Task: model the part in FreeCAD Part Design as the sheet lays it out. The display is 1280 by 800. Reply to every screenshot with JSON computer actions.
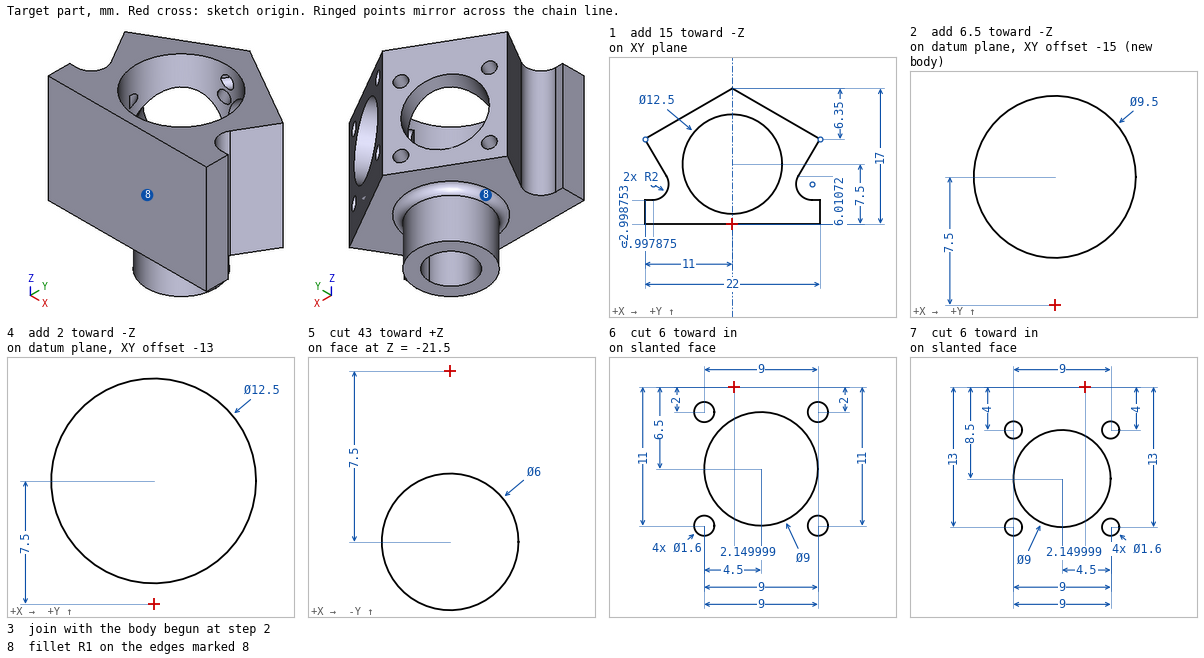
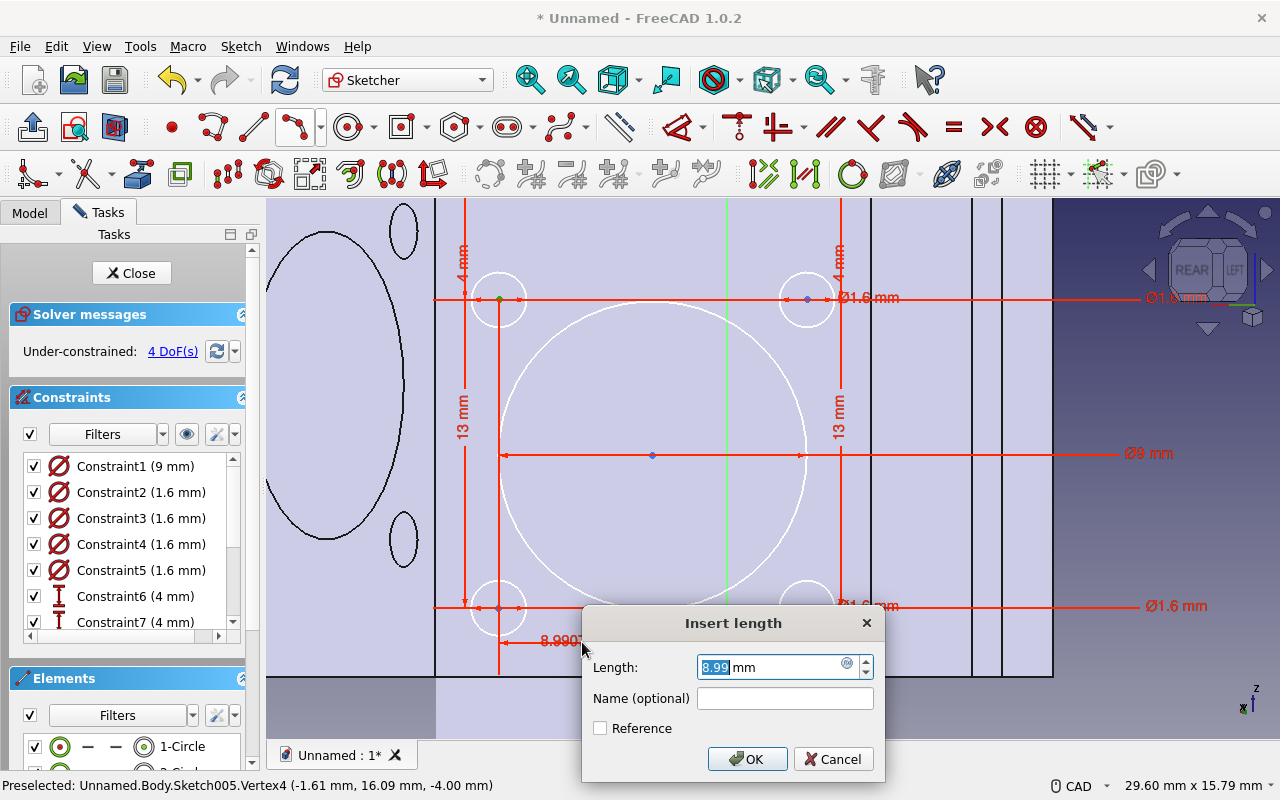
{"action": "type", "text": "9"}
{"action": "key", "text": "Return"}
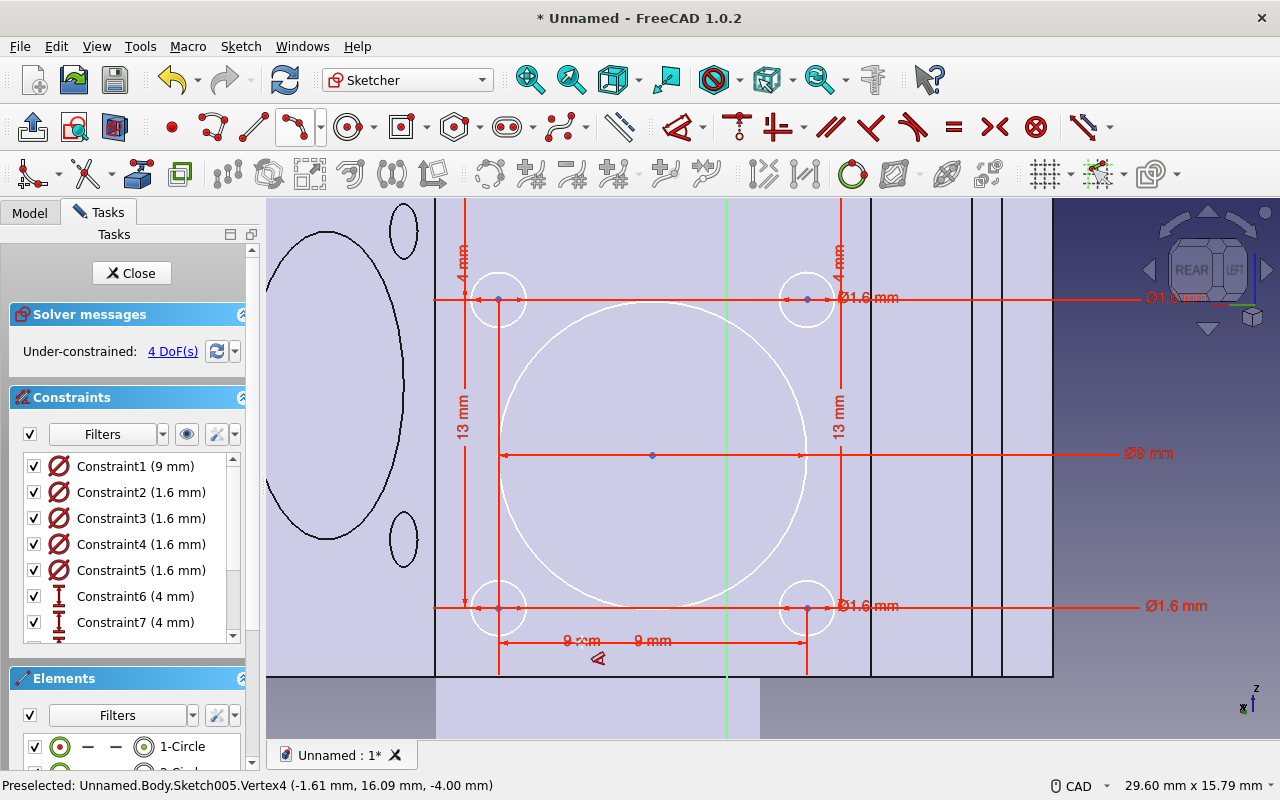
{"action": "left_click", "coordinate": [499, 300]}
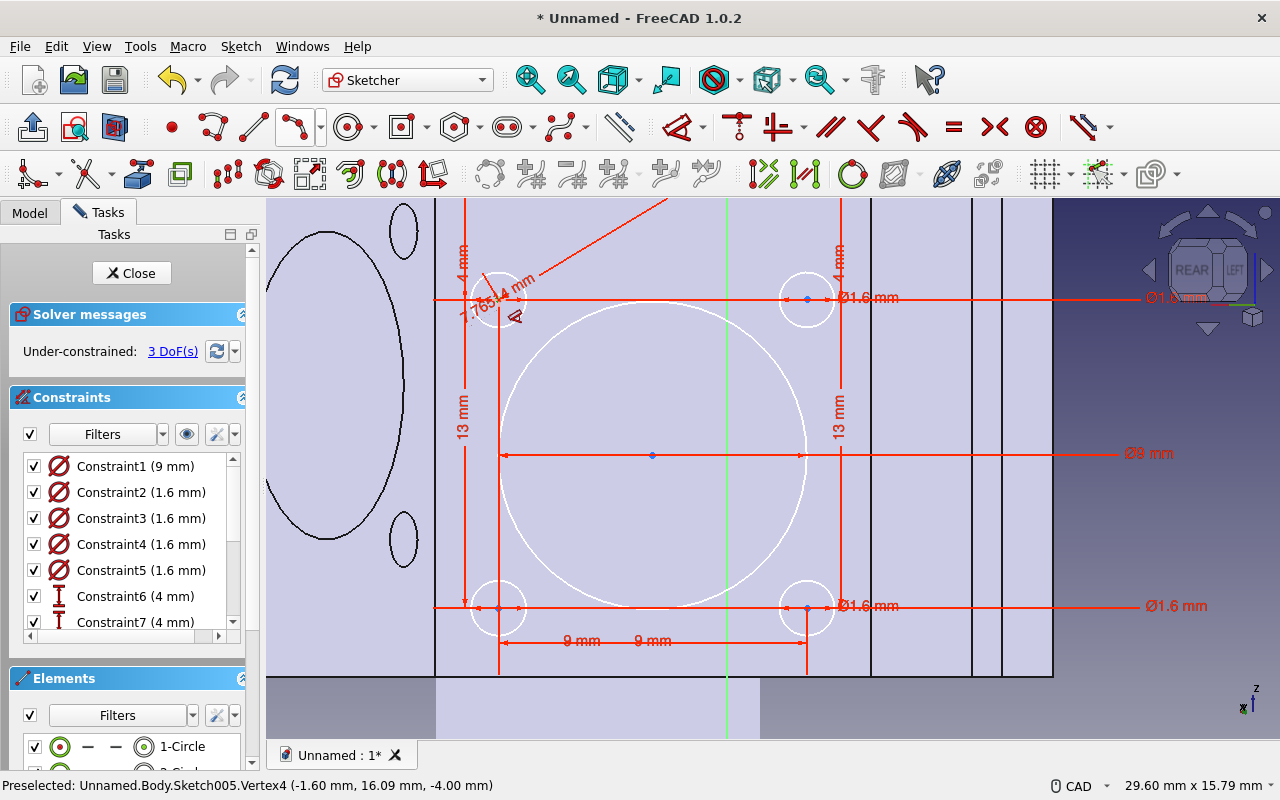
{"action": "left_click", "coordinate": [807, 300]}
{"action": "left_click", "coordinate": [653, 266]}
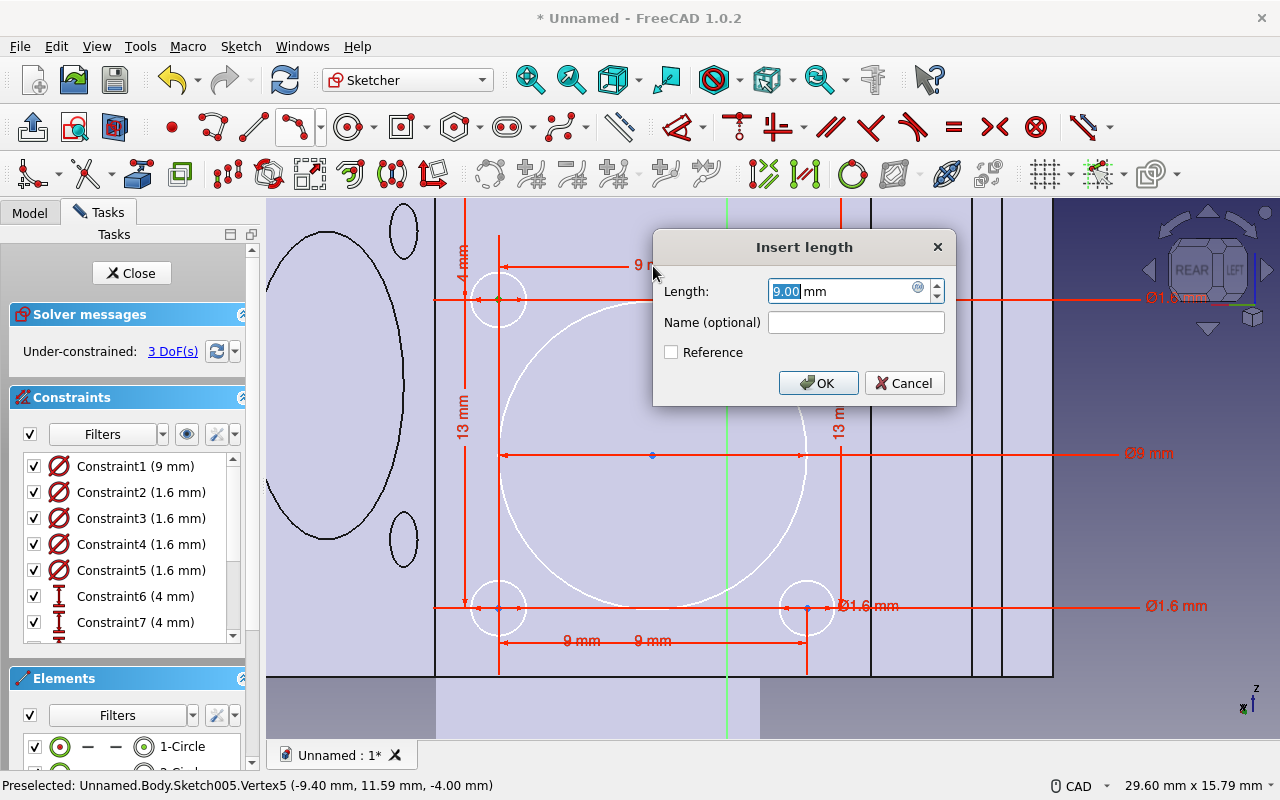
{"action": "type", "text": "9"}
{"action": "key", "text": "Return"}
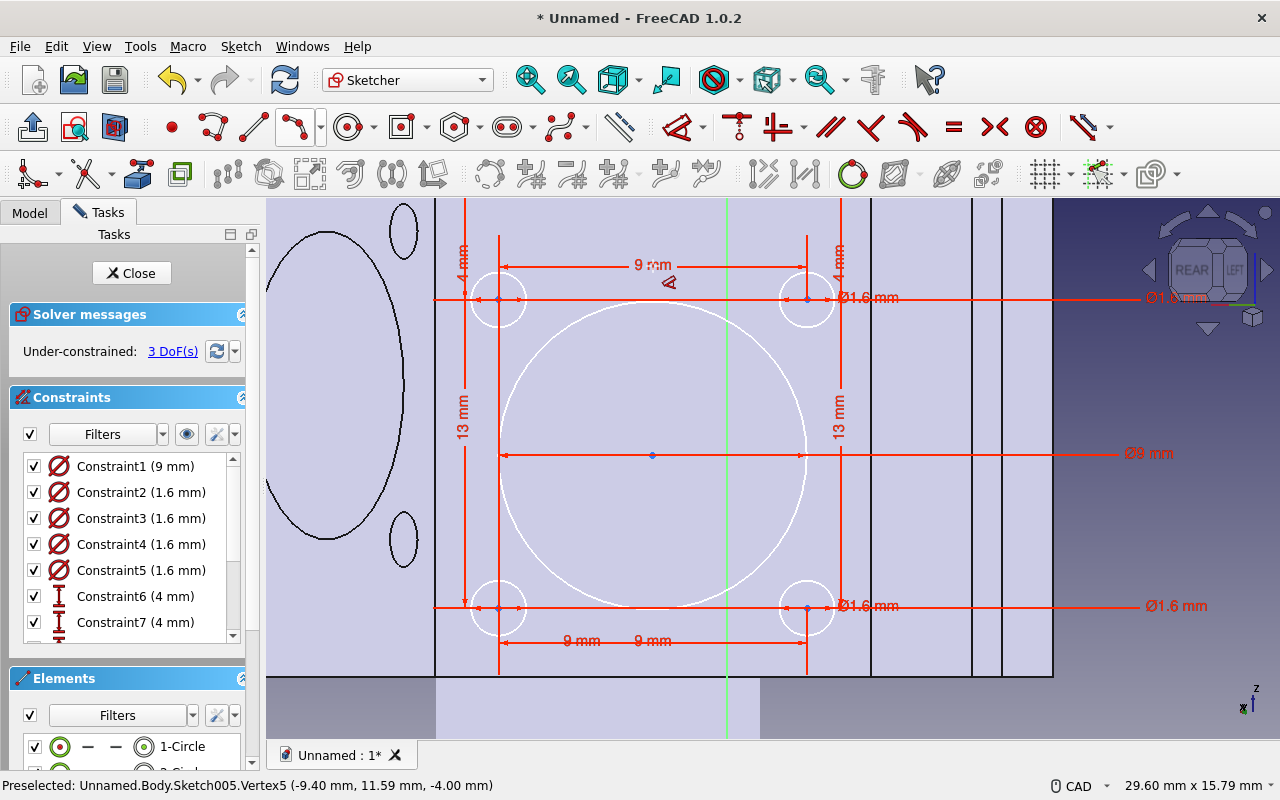
{"action": "left_click", "coordinate": [653, 455]}
{"action": "left_click", "coordinate": [761, 288]}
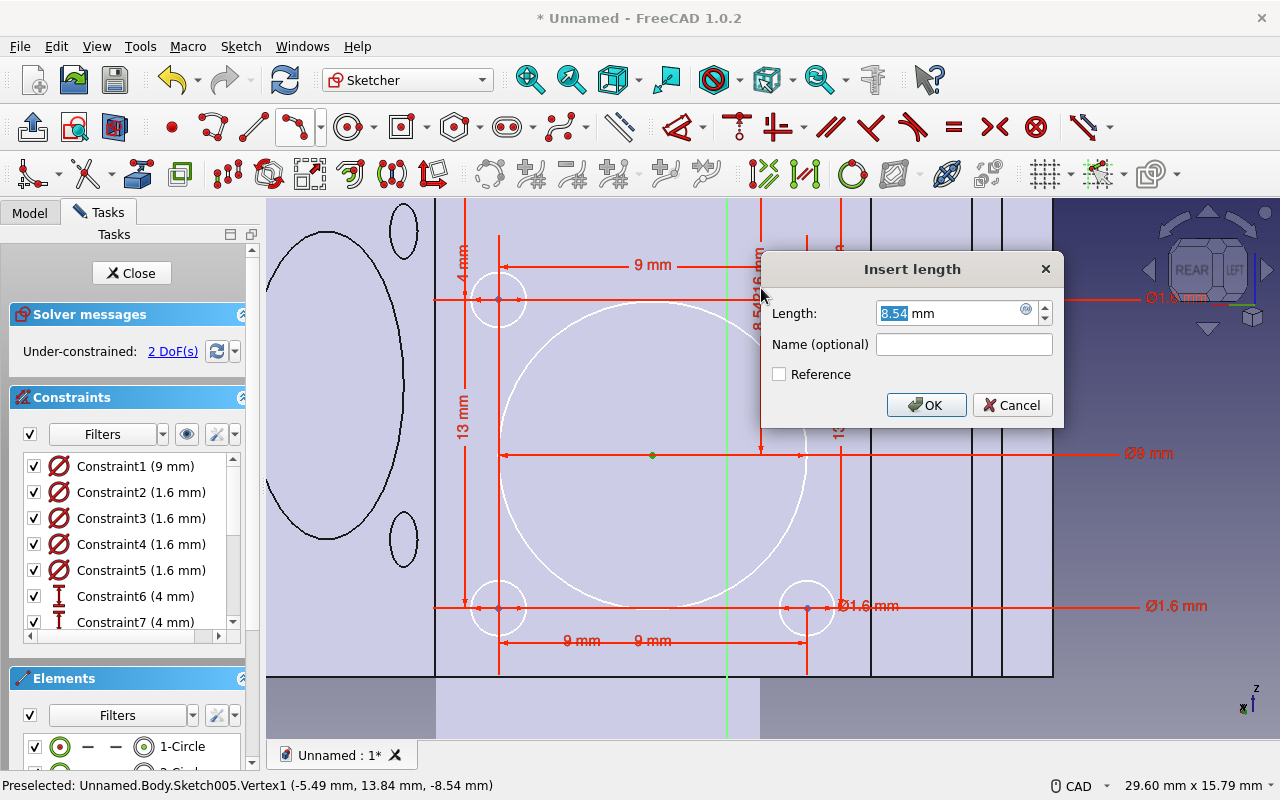
{"action": "type", "text": "8.5"}
{"action": "key", "text": "Return"}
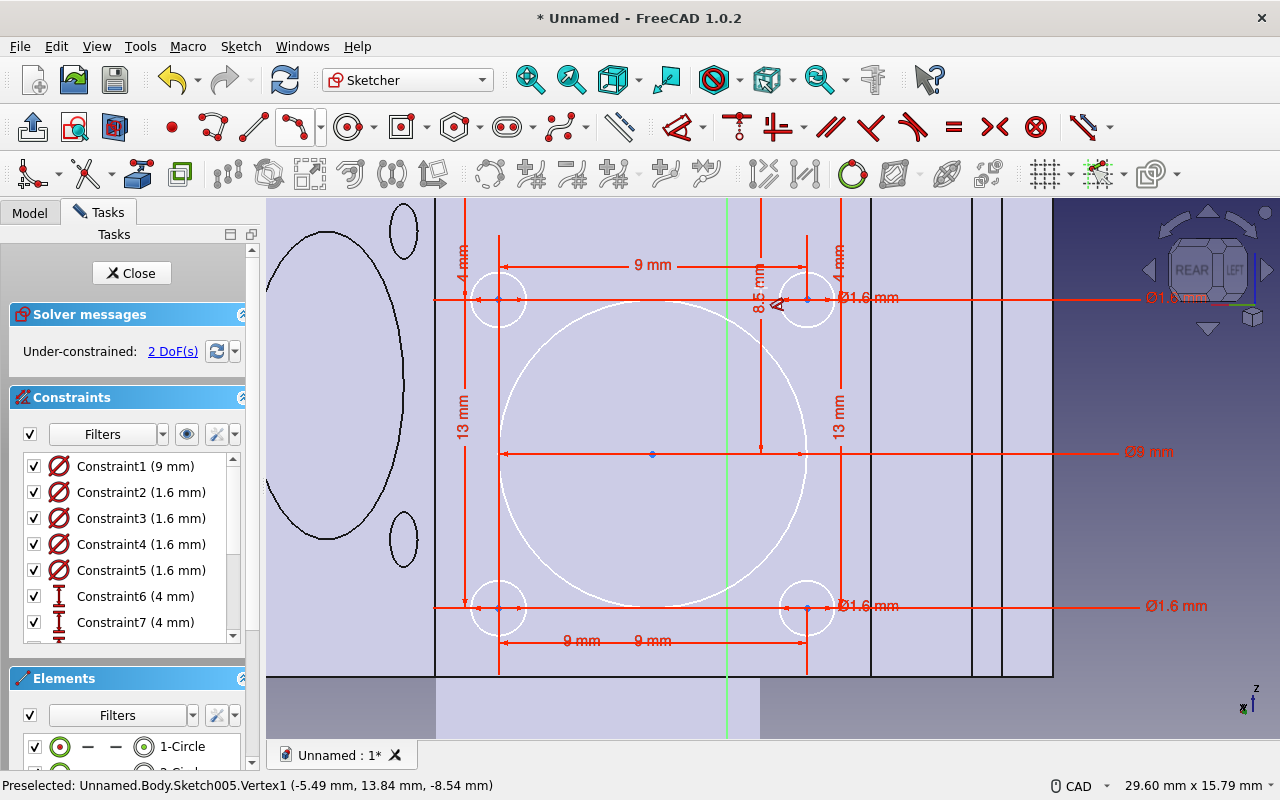
{"action": "left_click", "coordinate": [653, 454]}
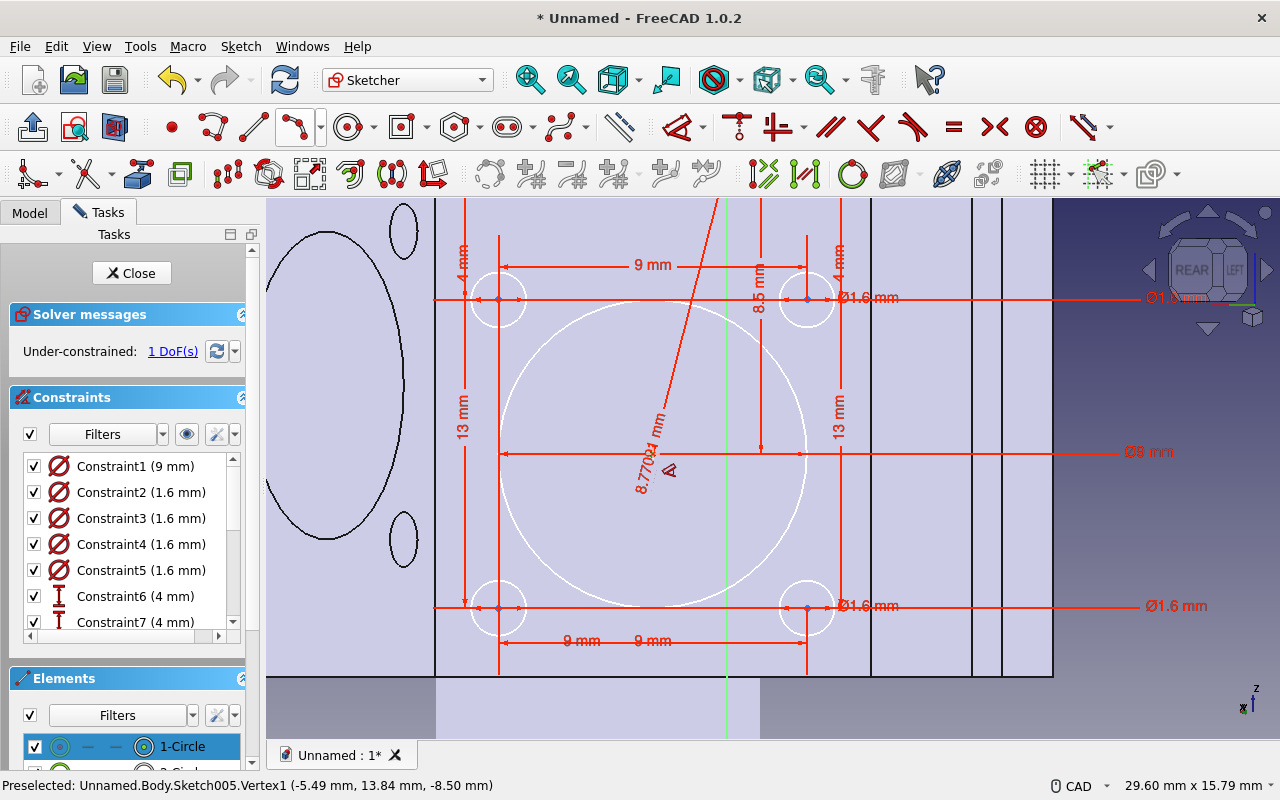
{"action": "left_click", "coordinate": [807, 608]}
{"action": "left_click", "coordinate": [765, 642]}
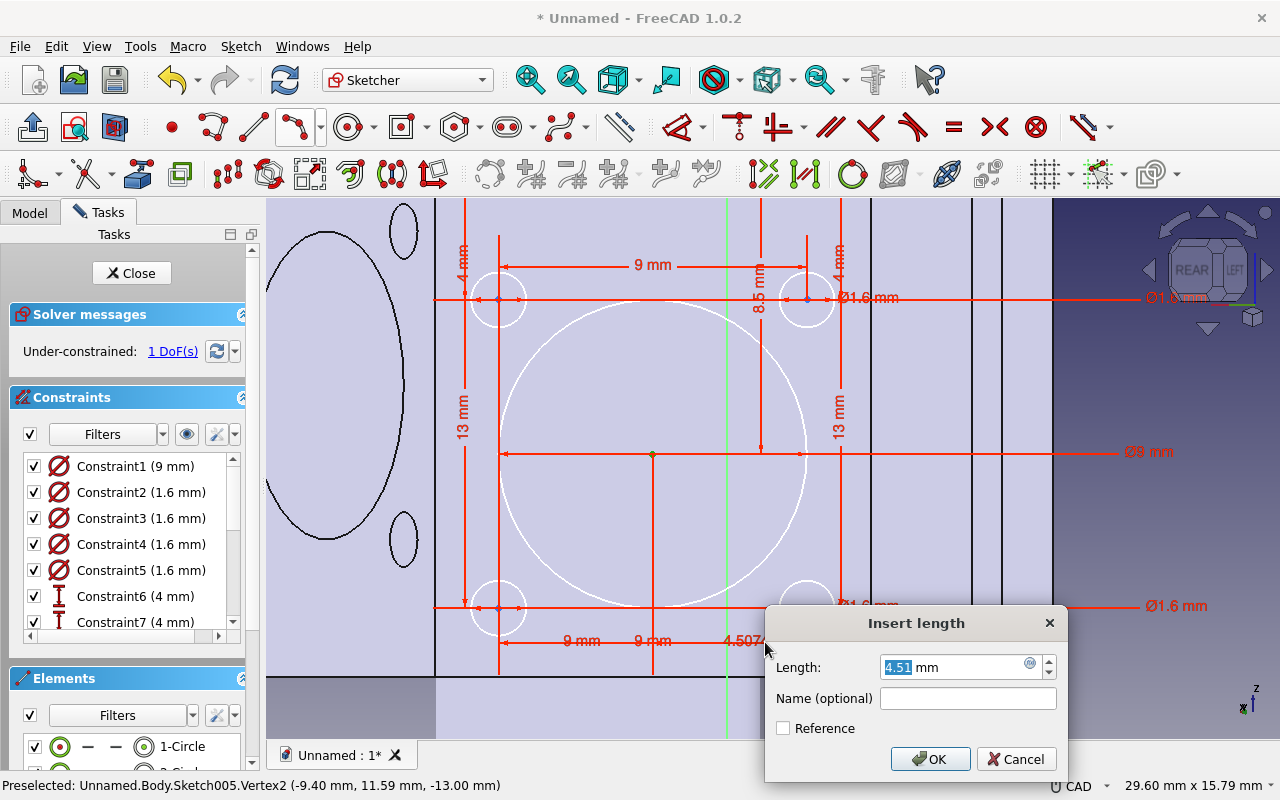
{"action": "type", "text": "4.5"}
{"action": "key", "text": "Return"}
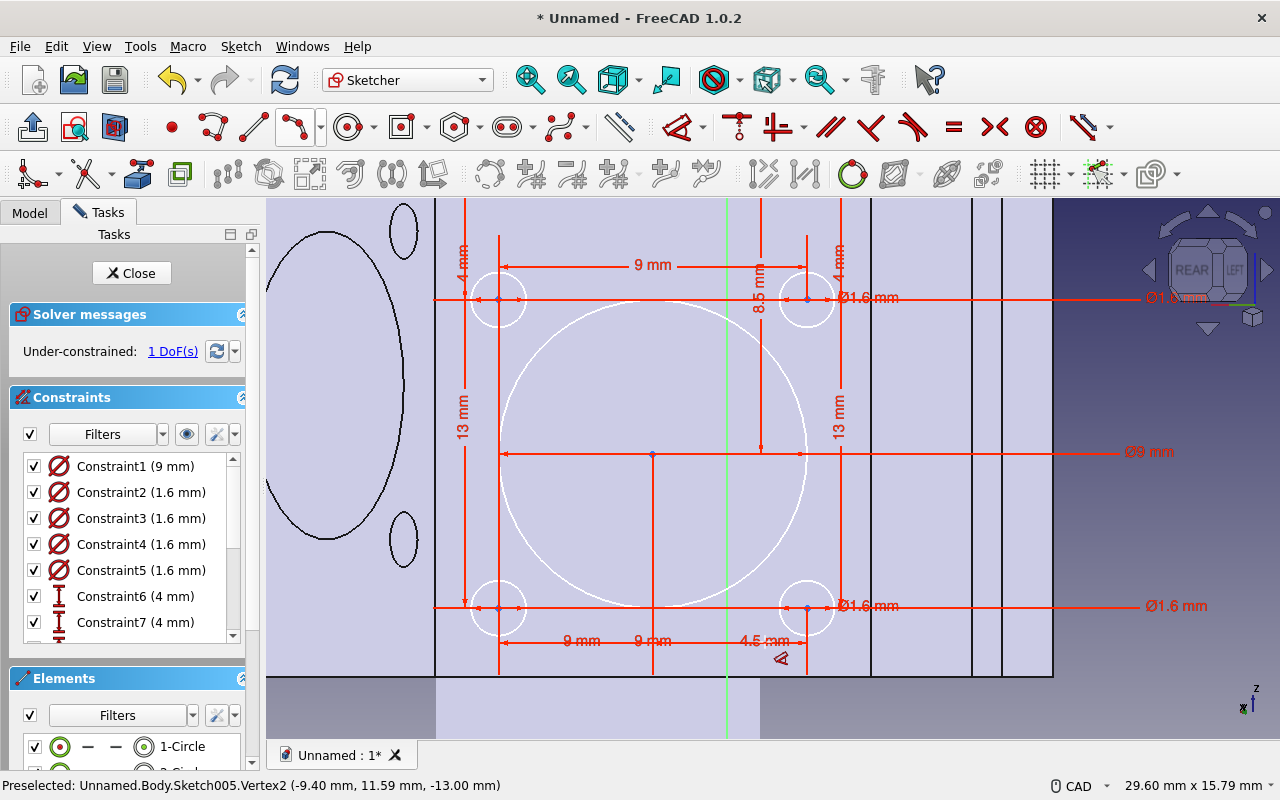
{"action": "left_click", "coordinate": [653, 454]}
{"action": "left_click", "coordinate": [690, 488]}